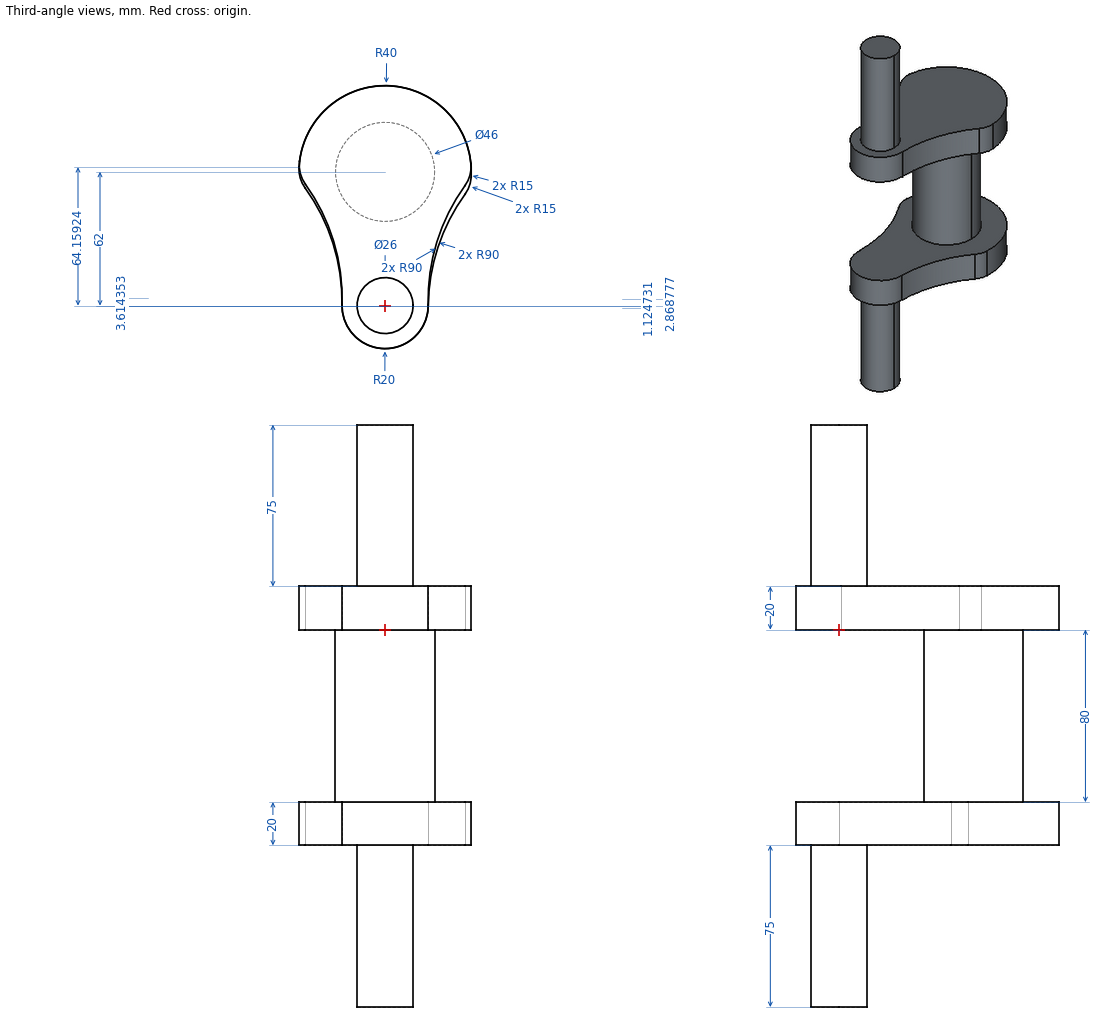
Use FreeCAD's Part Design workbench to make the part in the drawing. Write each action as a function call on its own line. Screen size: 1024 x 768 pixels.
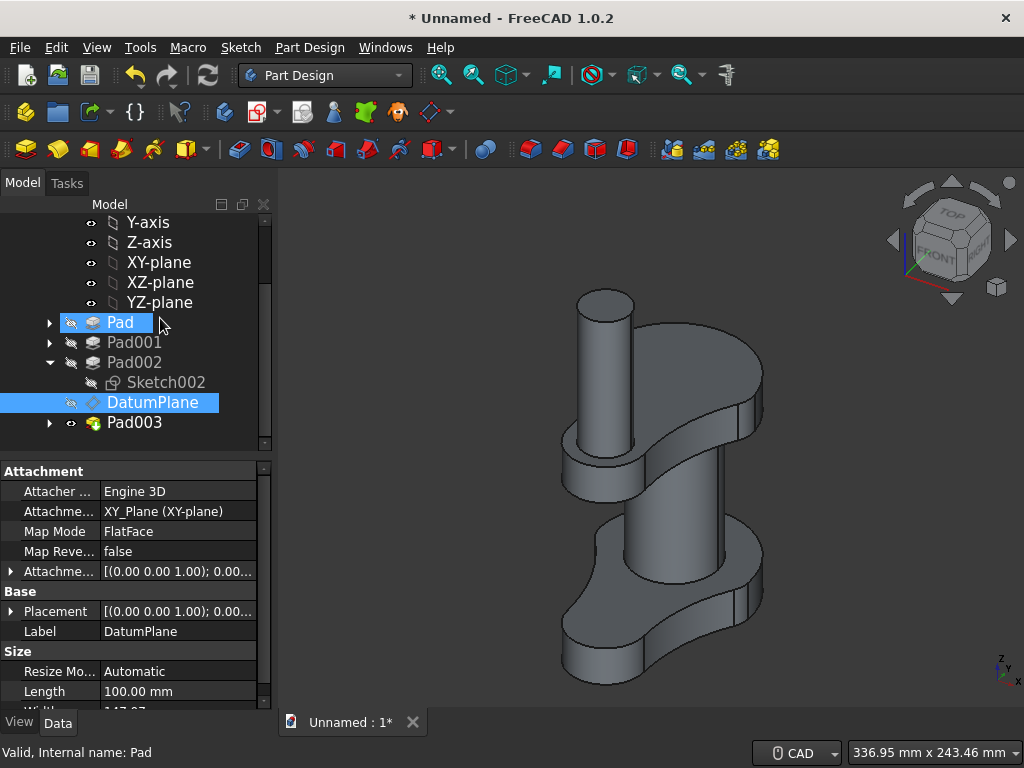
scroll(160, 318, up, 15)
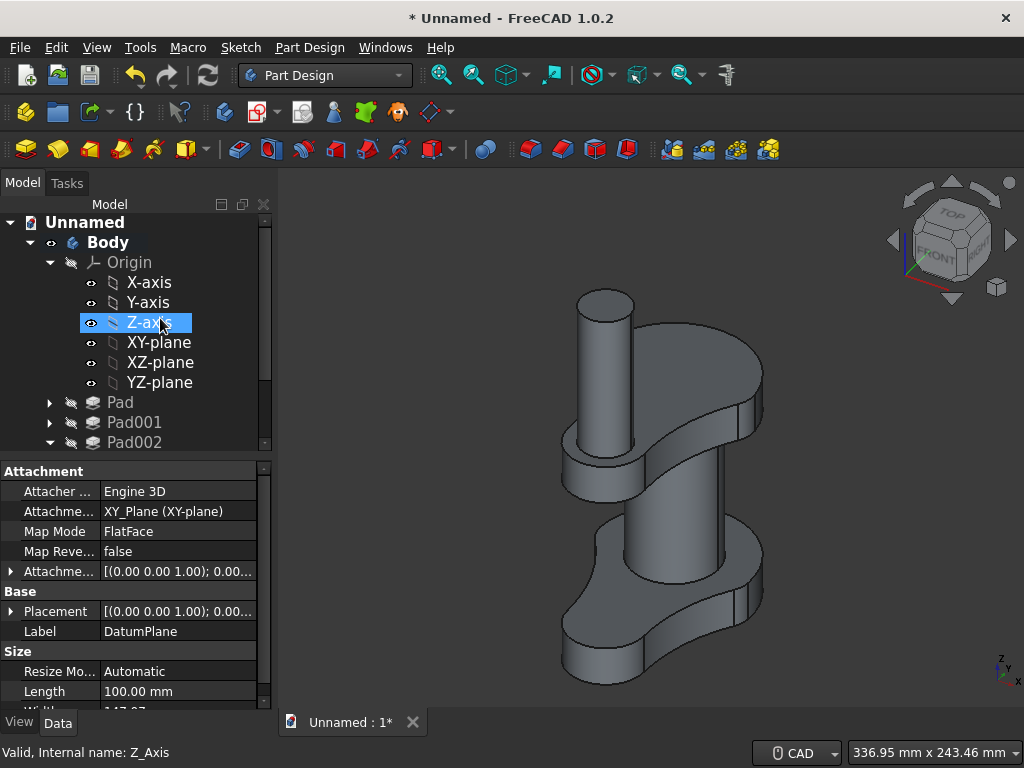
click(136, 343)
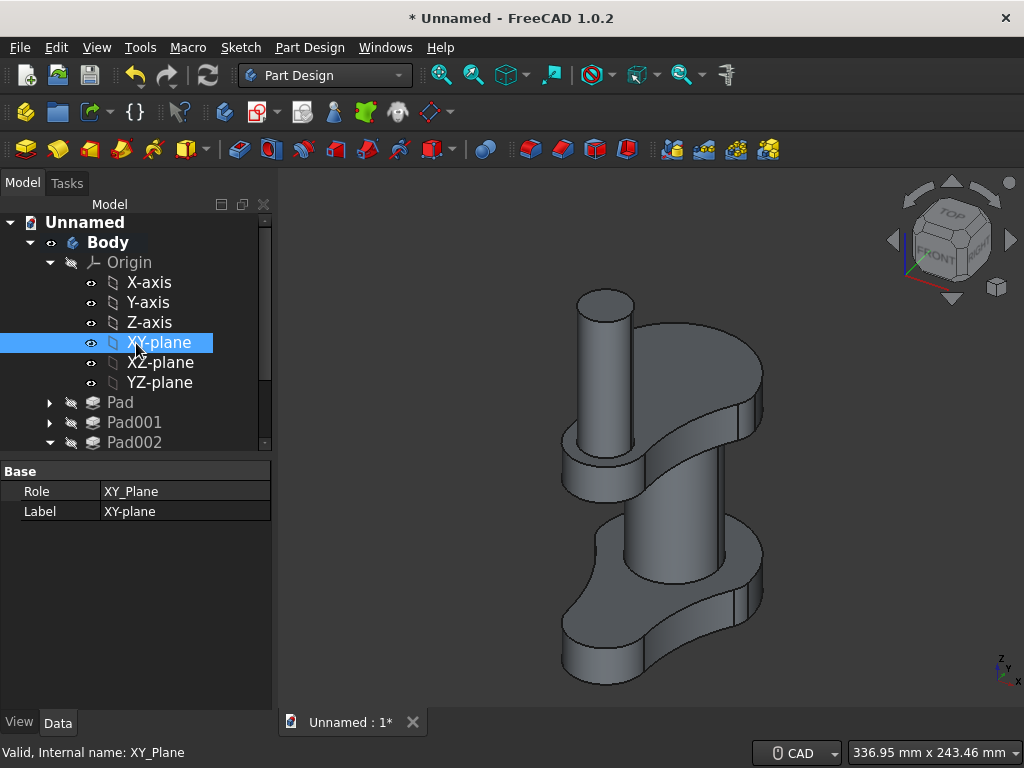
click(430, 112)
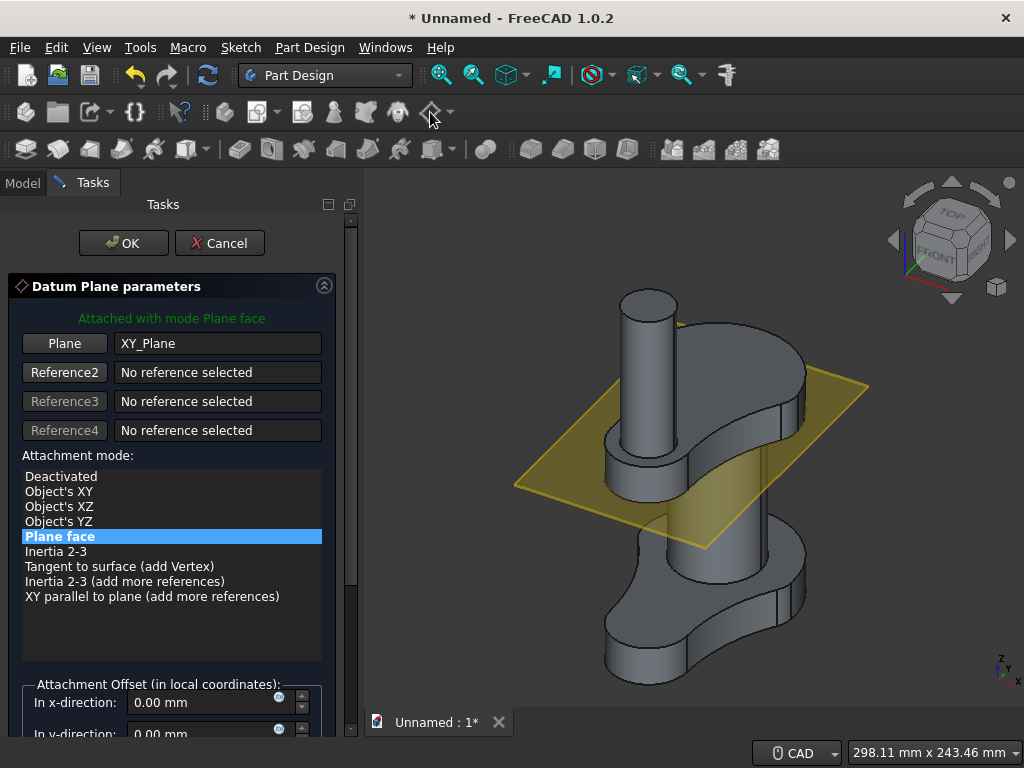
scroll(351, 475, down, 2)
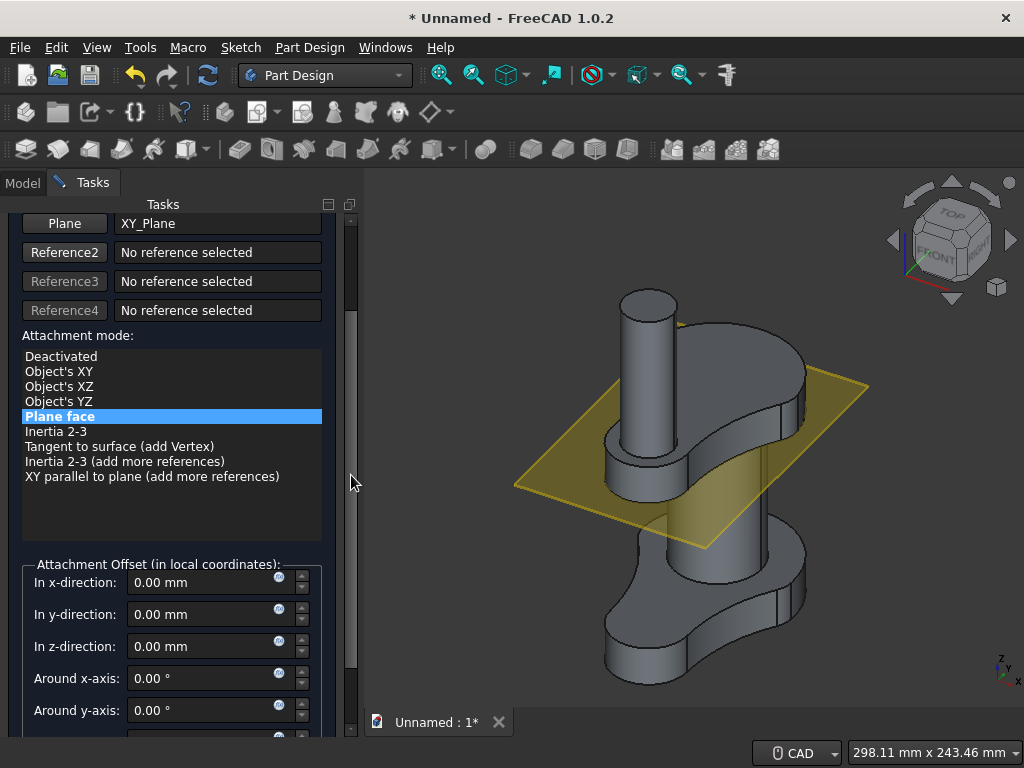
triple_click(210, 646)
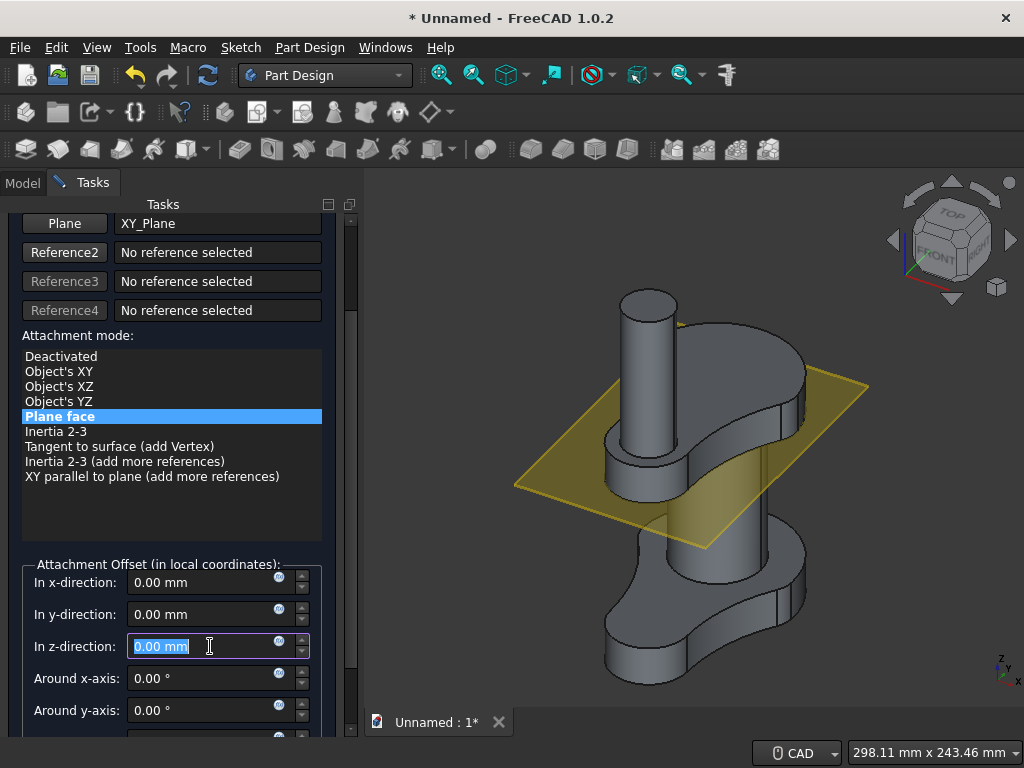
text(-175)
key(Tab)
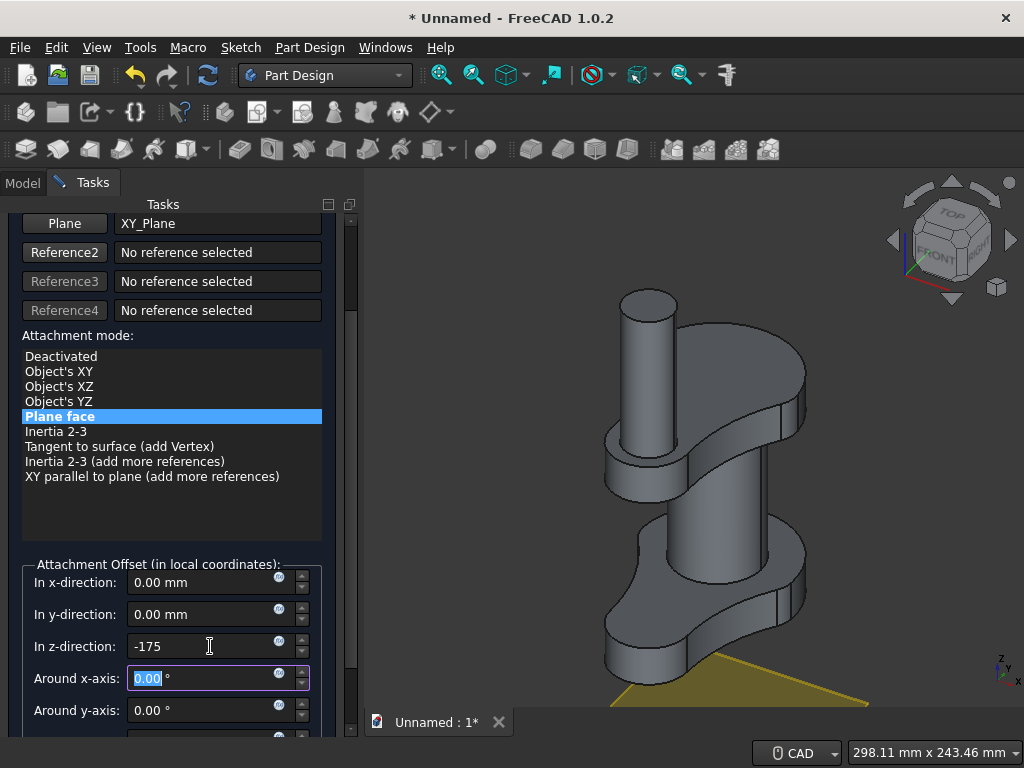
scroll(351, 475, up, 3)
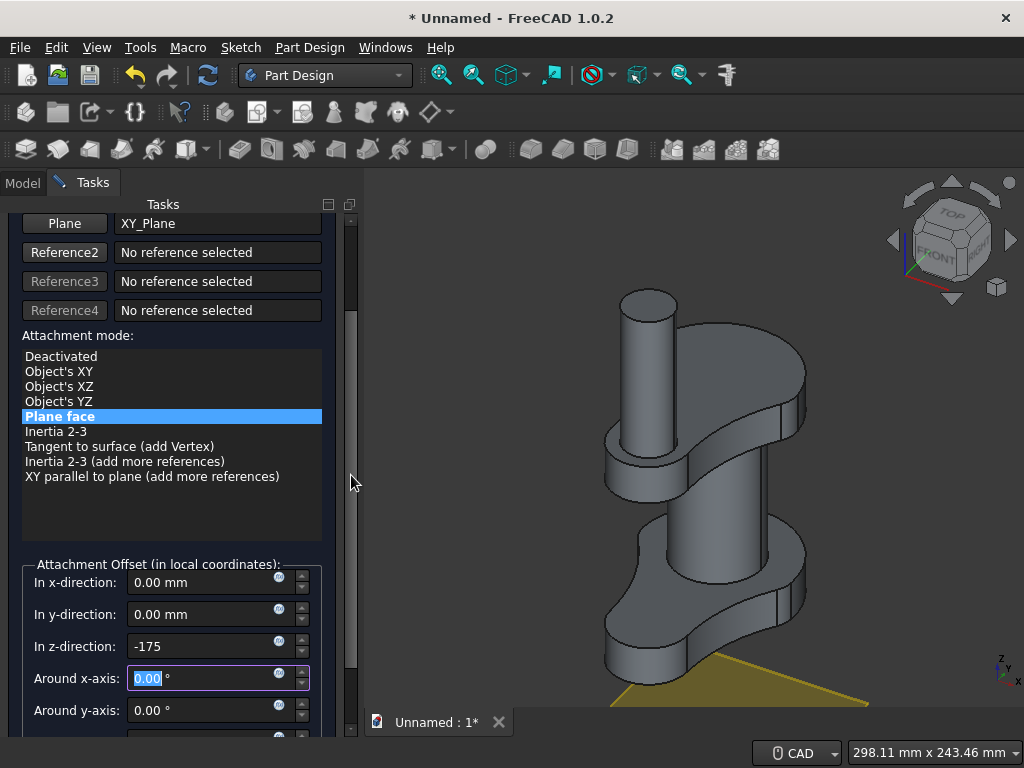
click(124, 243)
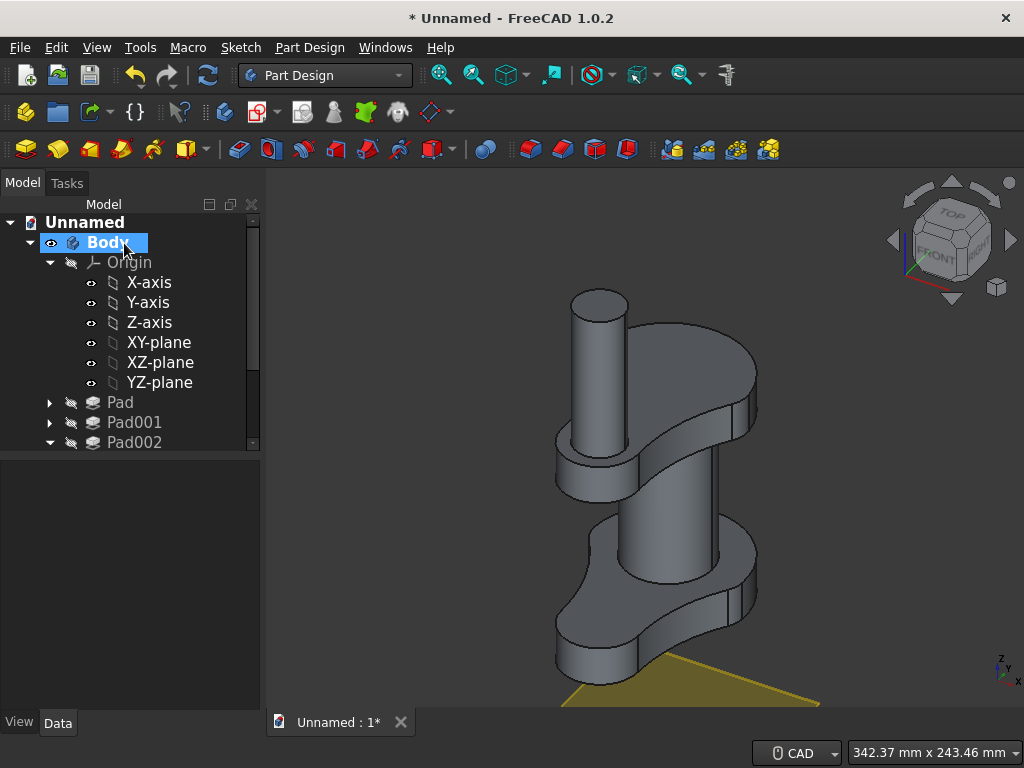
scroll(100, 338, down, 3)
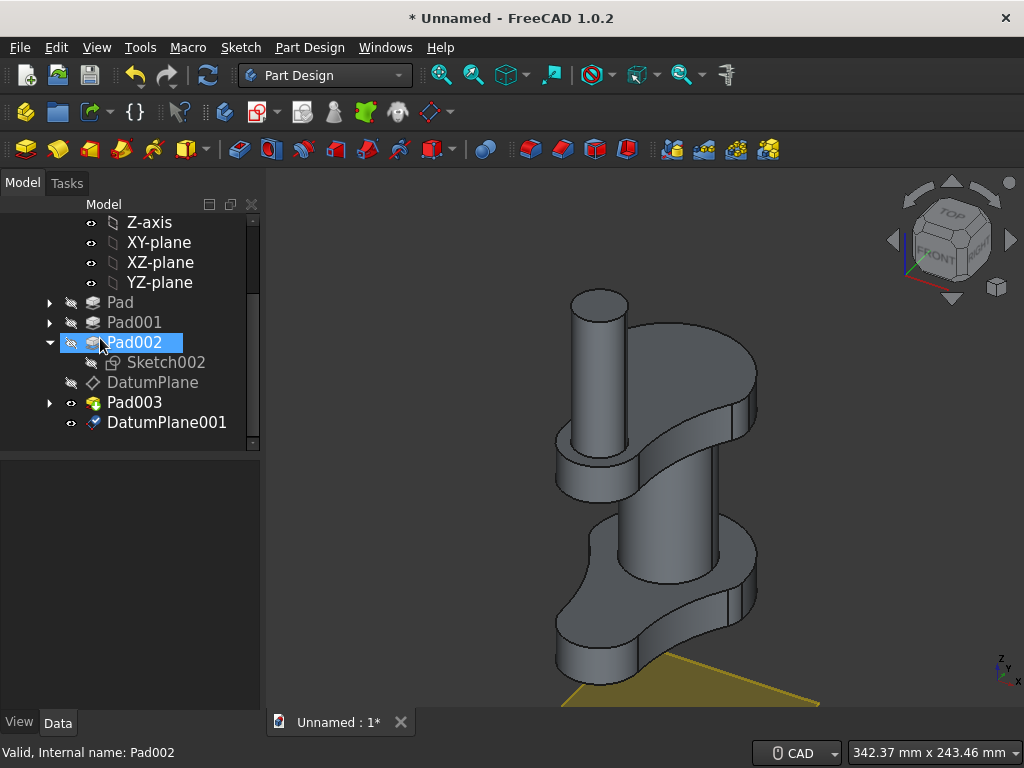
click(116, 423)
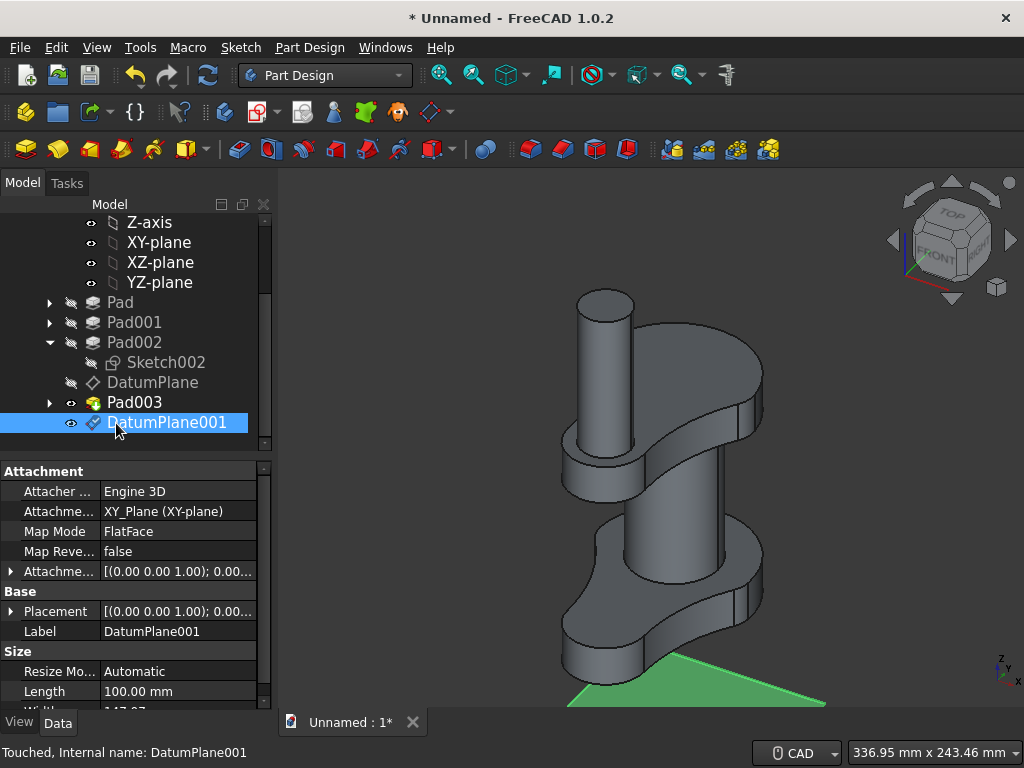
click(258, 112)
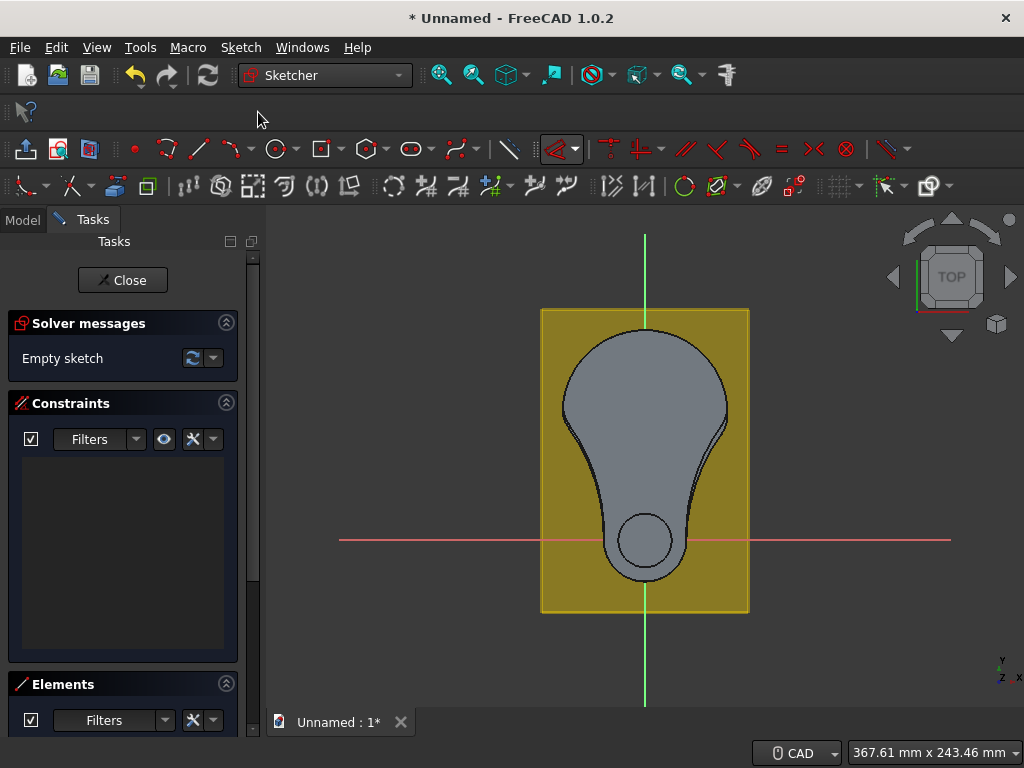
click(90, 150)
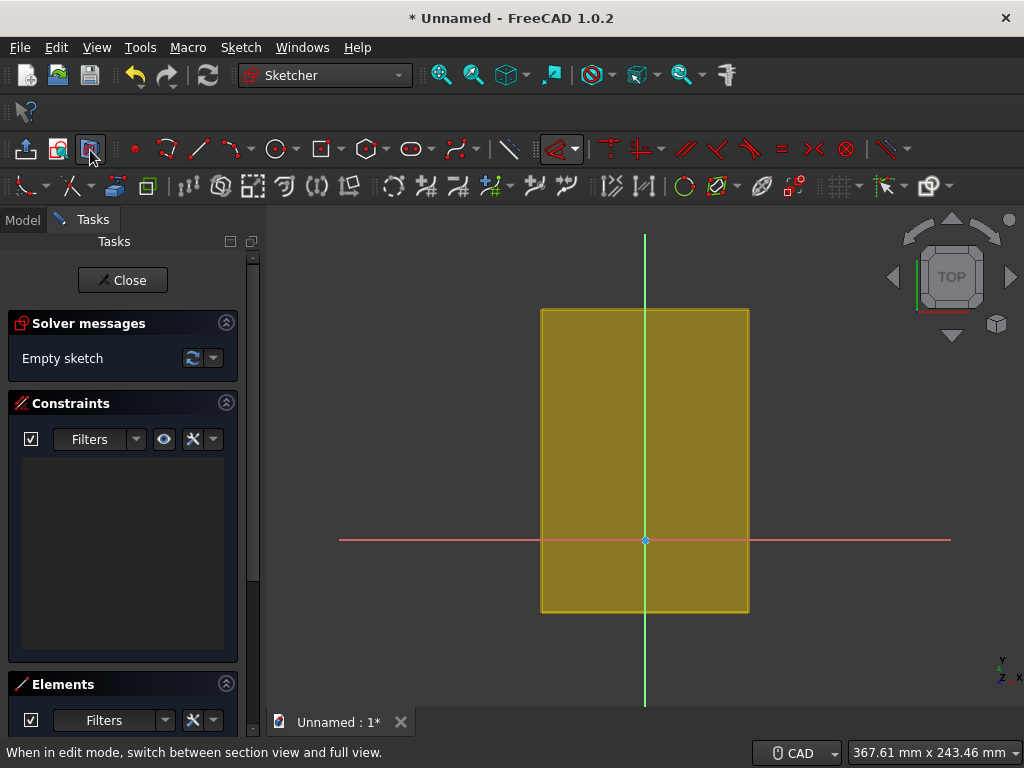
scroll(659, 557, up, 9)